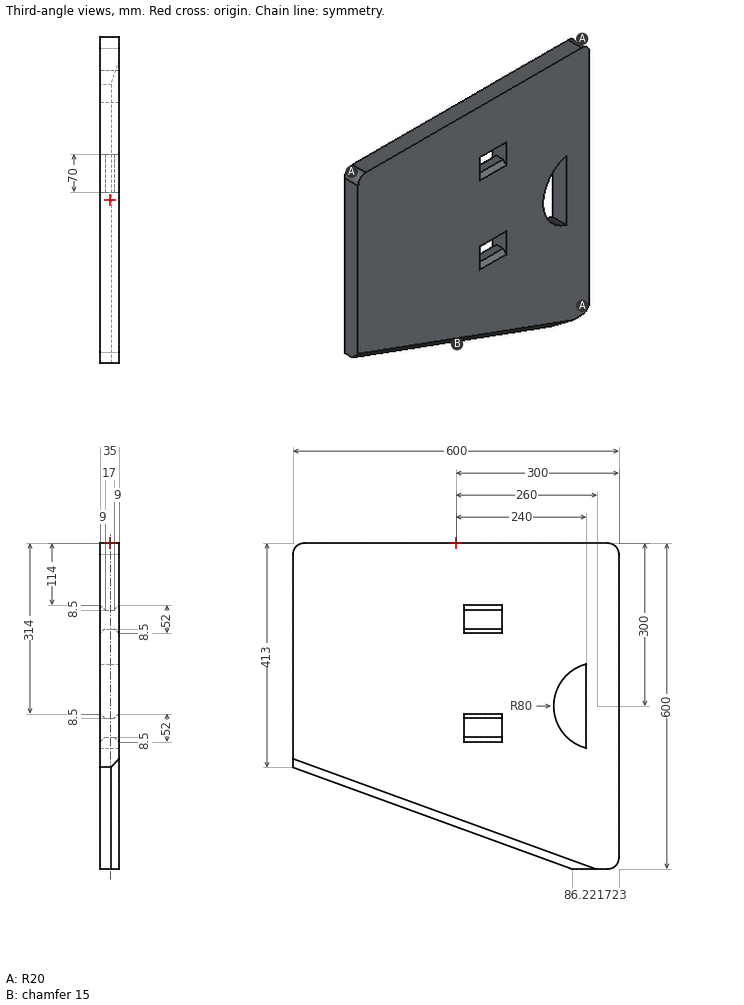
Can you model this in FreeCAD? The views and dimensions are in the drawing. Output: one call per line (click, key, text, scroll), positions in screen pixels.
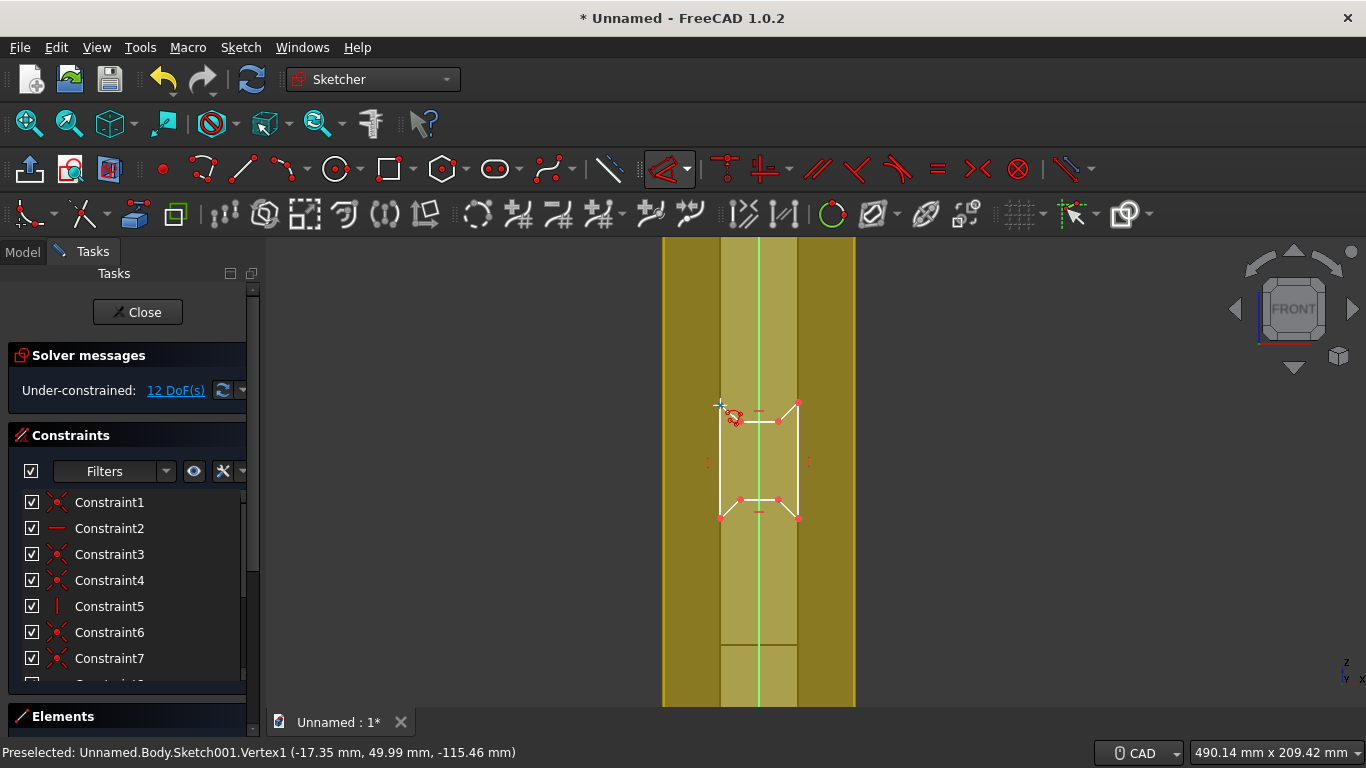
scroll(741, 423, down, 5)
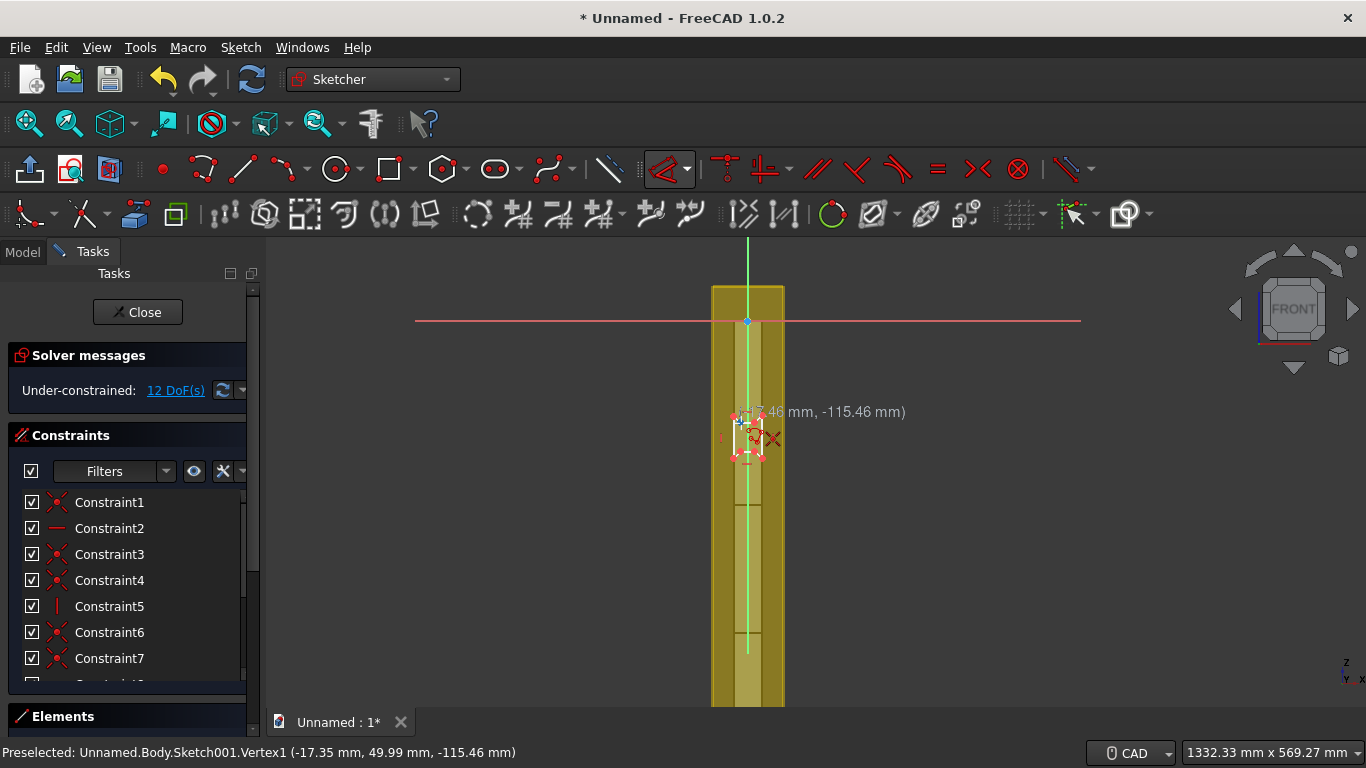
click(734, 581)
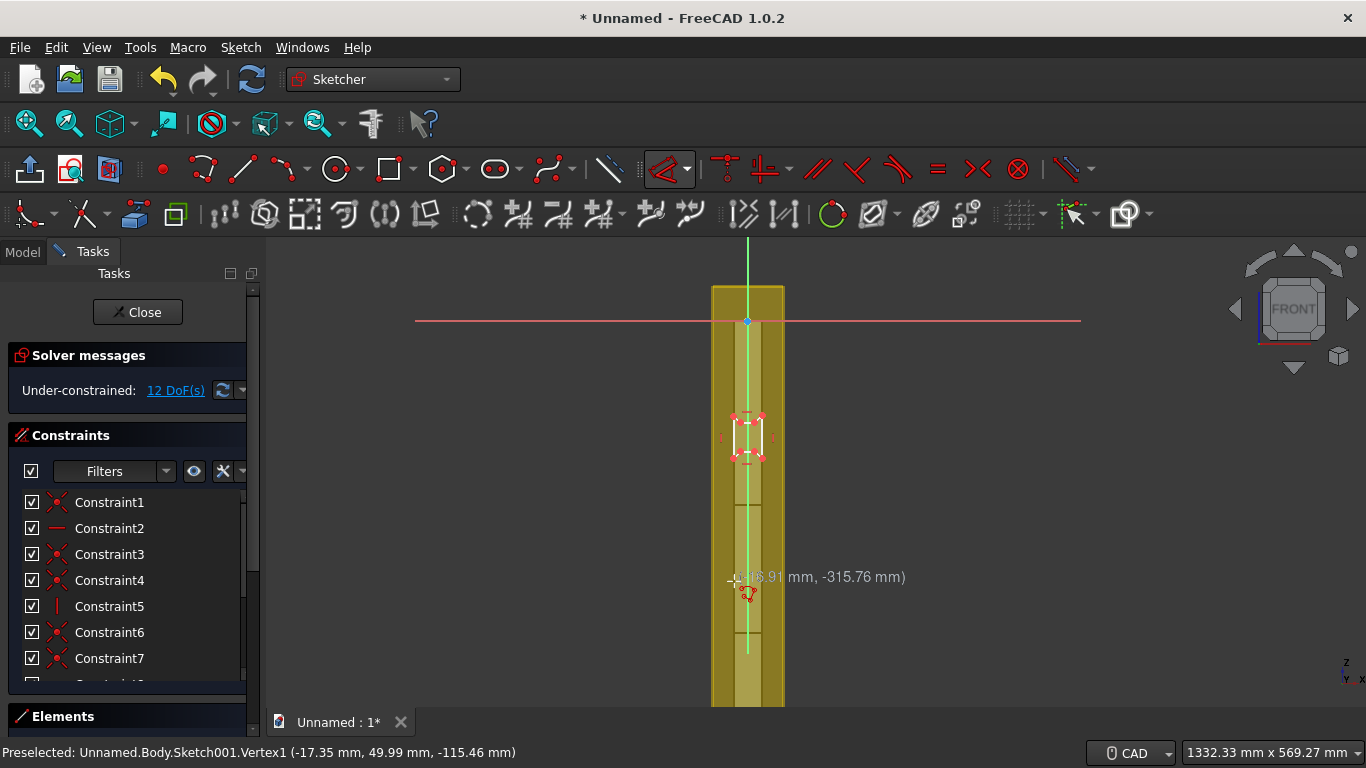
scroll(741, 588, up, 5)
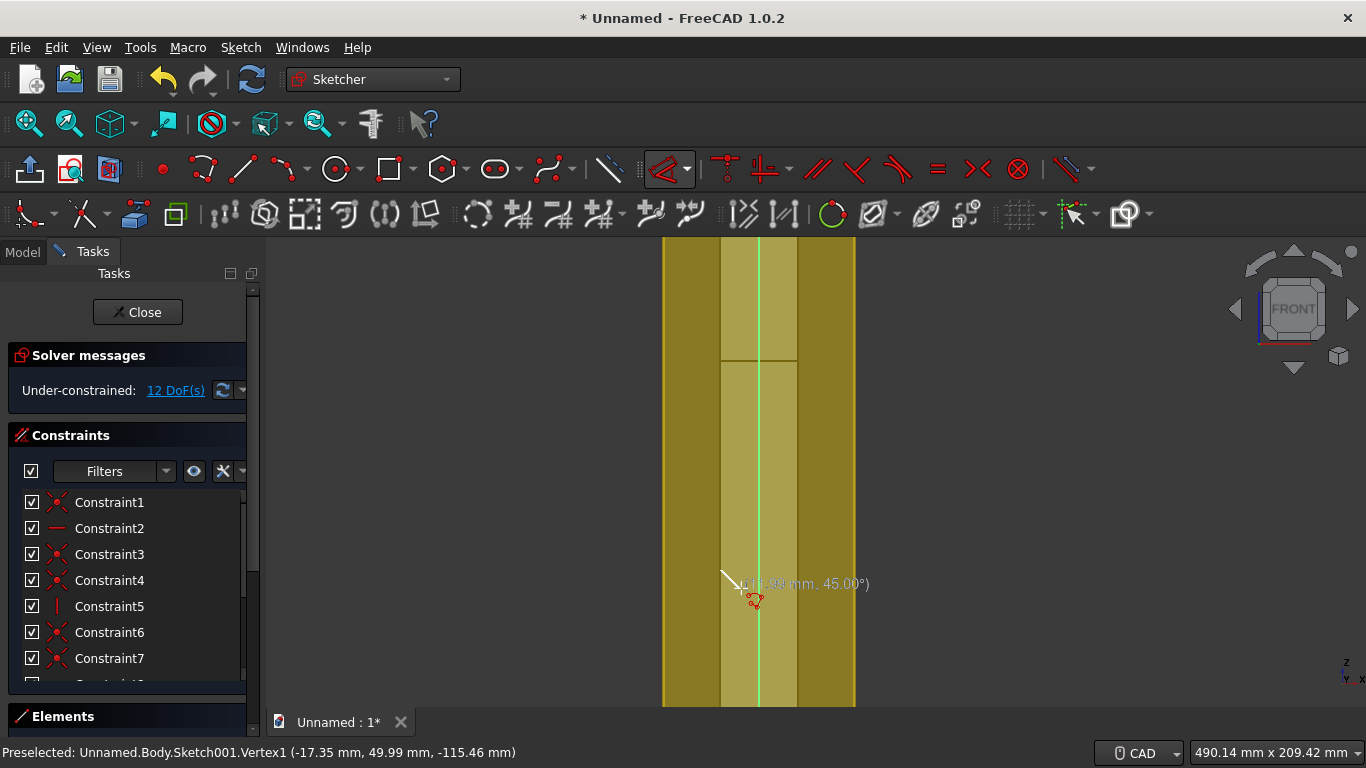
click(740, 586)
click(778, 586)
click(798, 566)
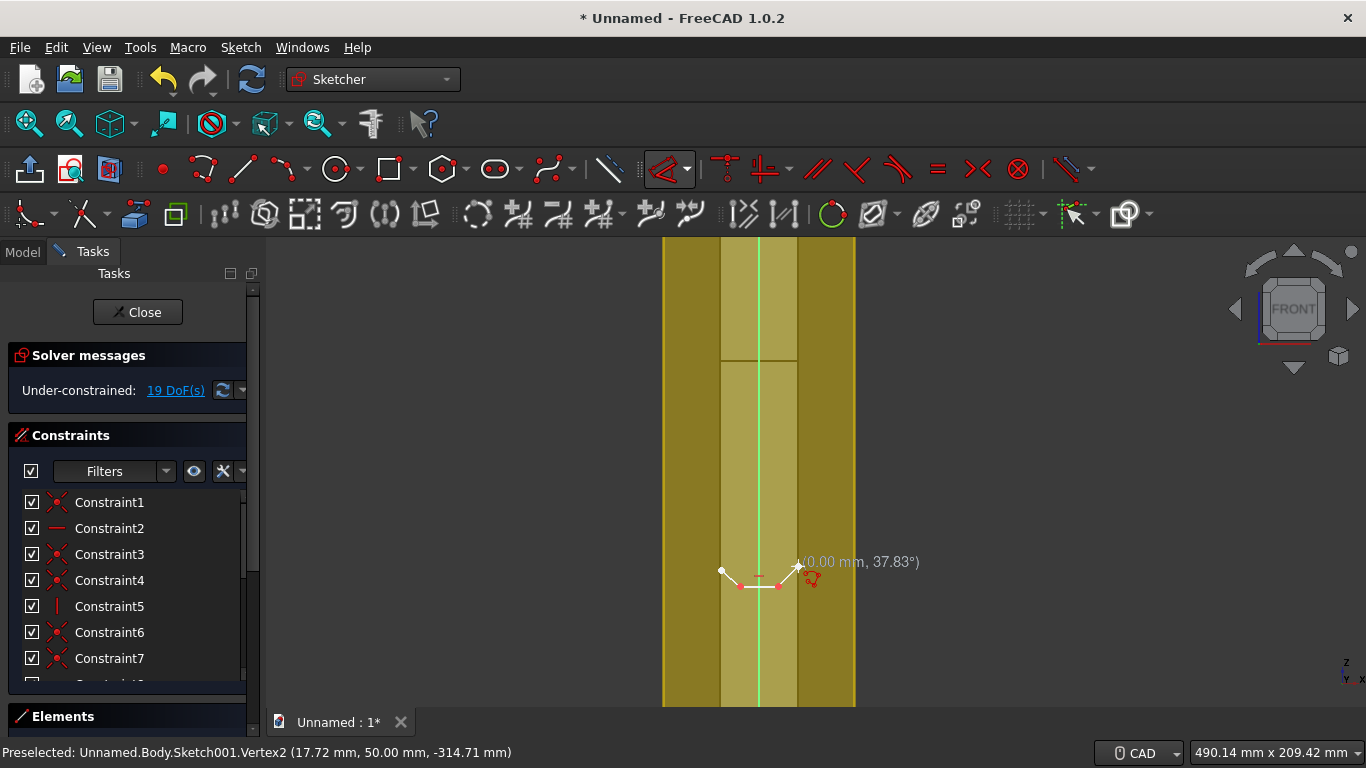
scroll(741, 588, down, 5)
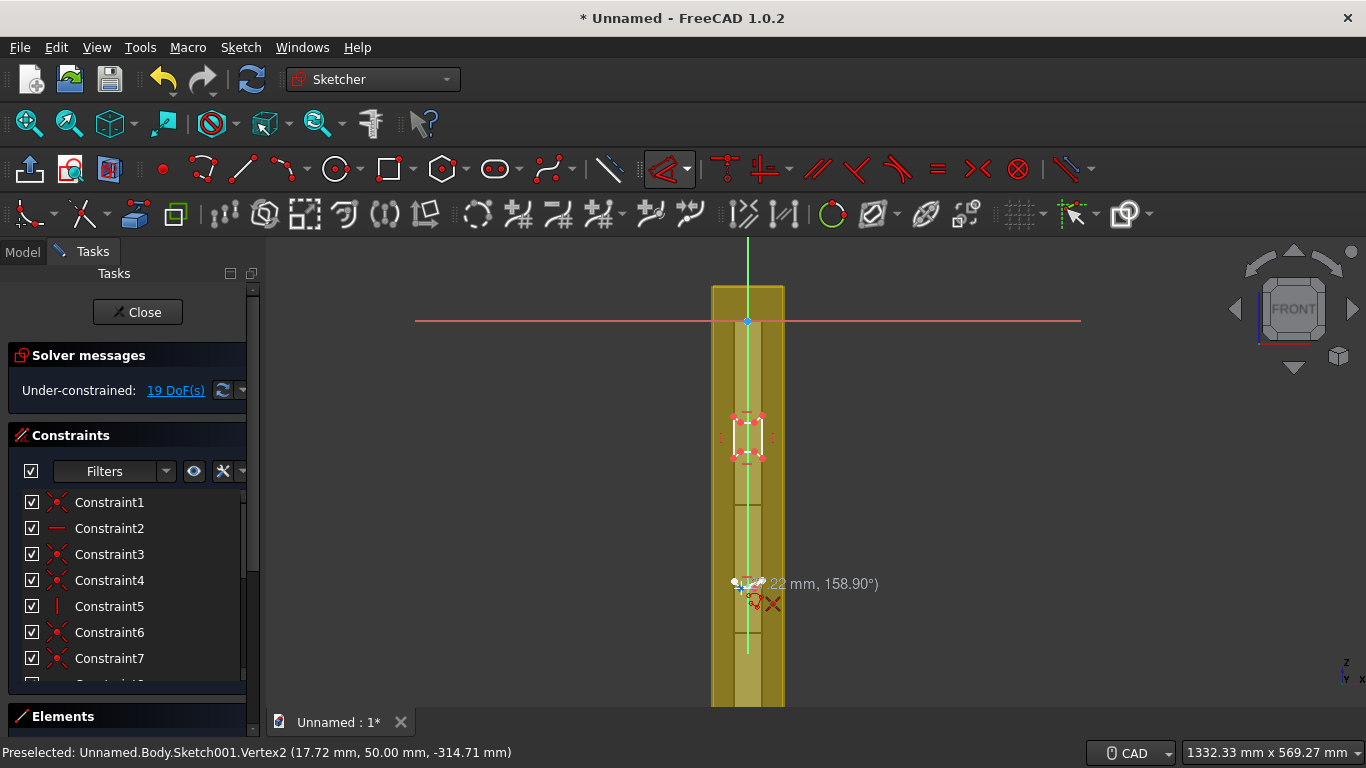
click(762, 623)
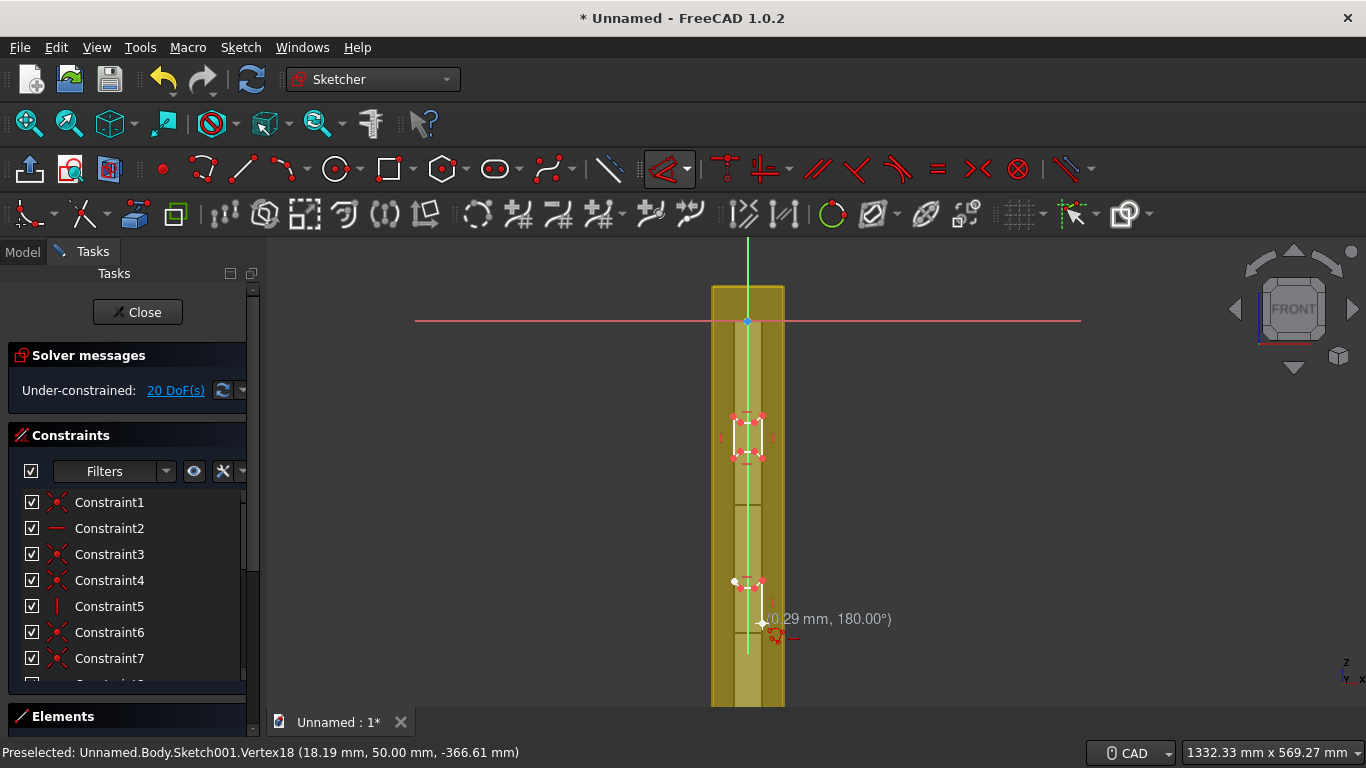
scroll(755, 616, up, 5)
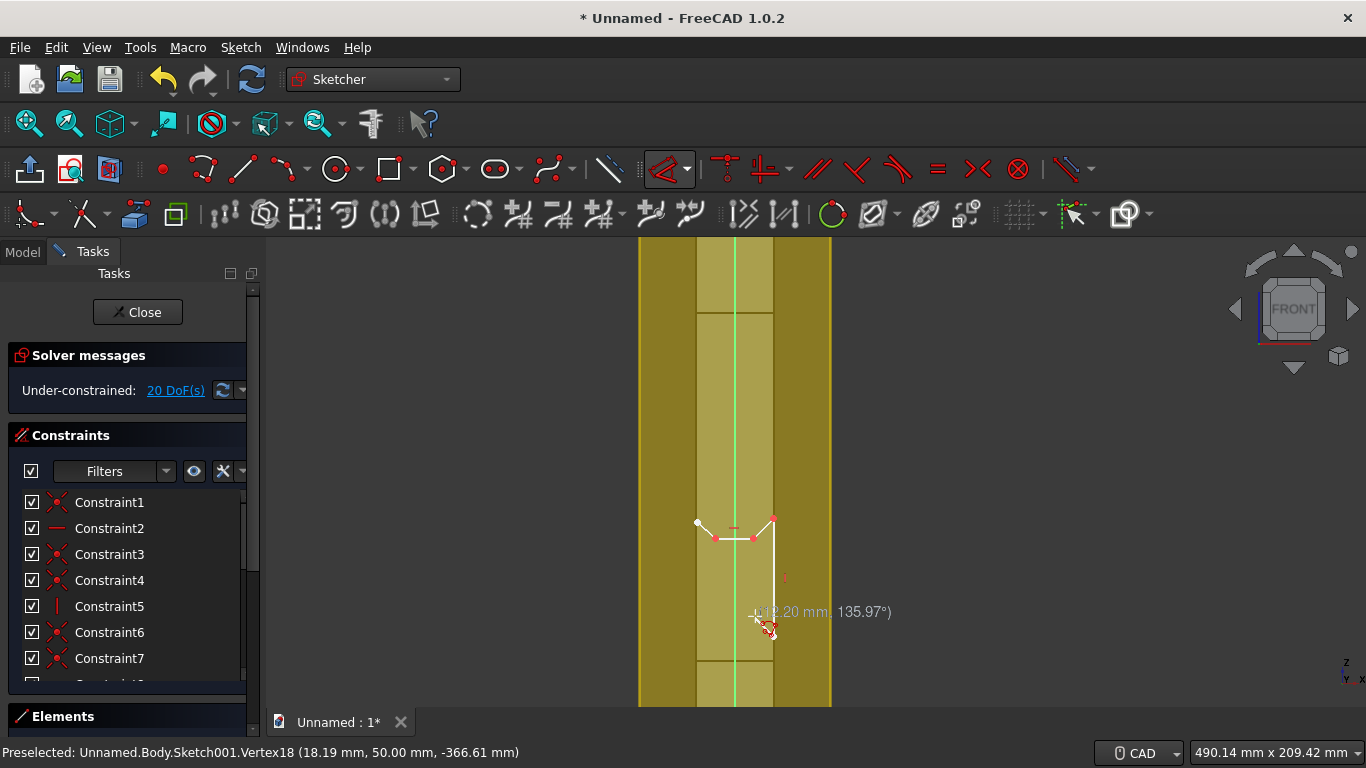
click(754, 616)
click(716, 616)
click(696, 635)
click(697, 522)
key(Escape)
key(Escape)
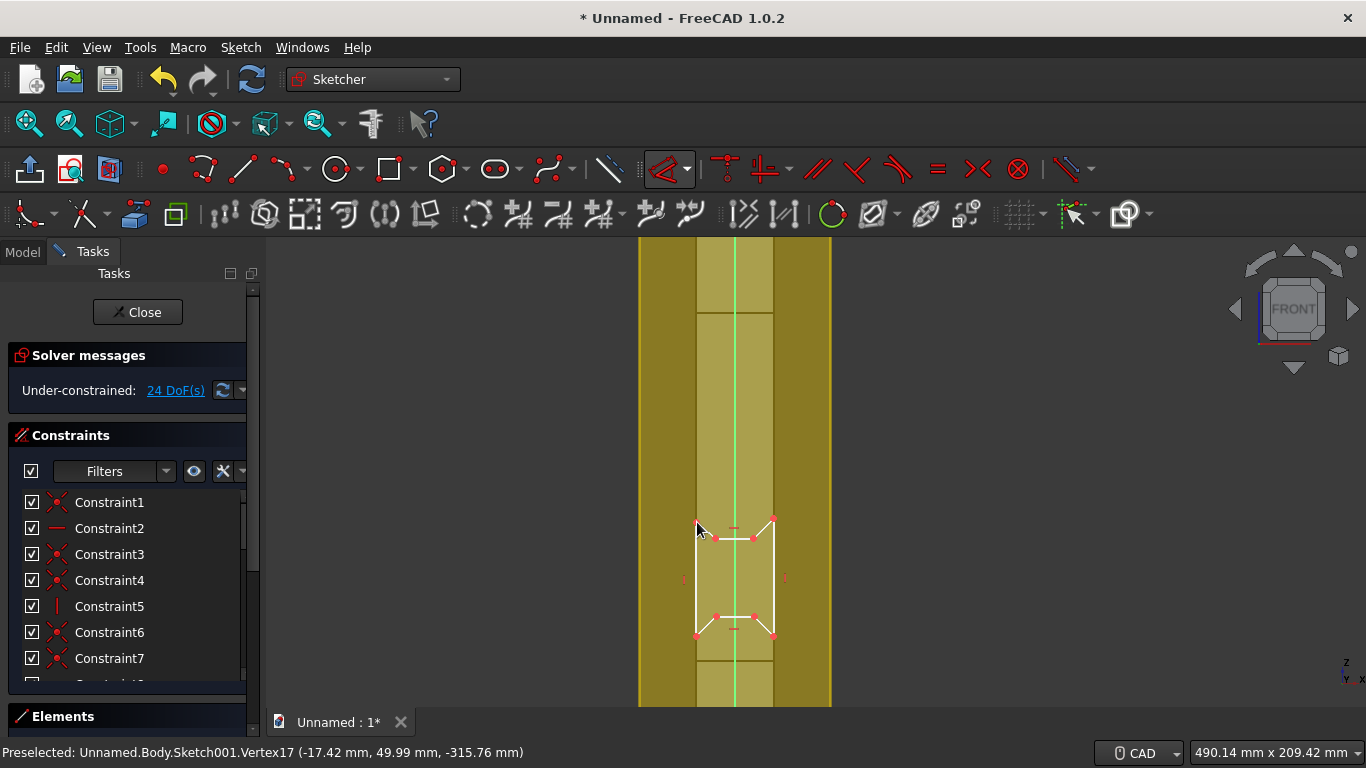
scroll(755, 616, down, 5)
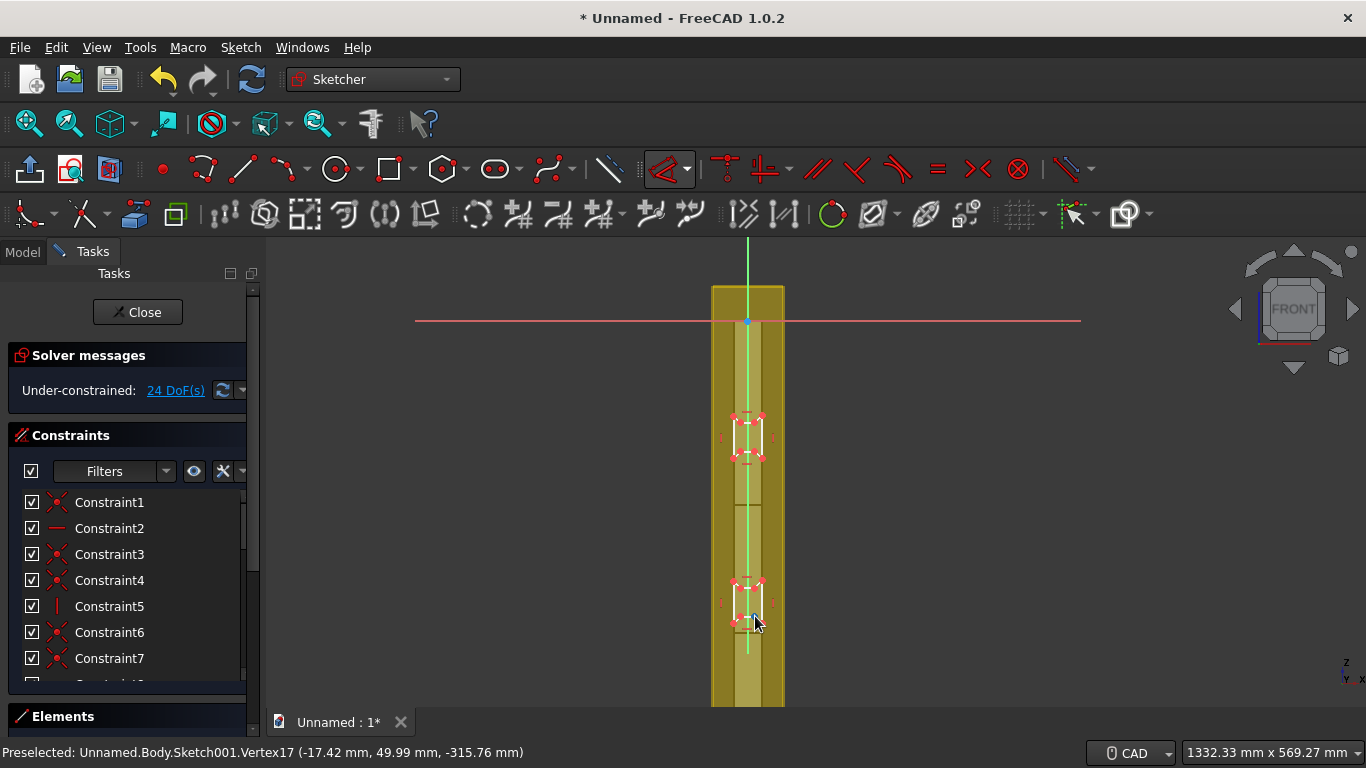
scroll(734, 417, up, 2)